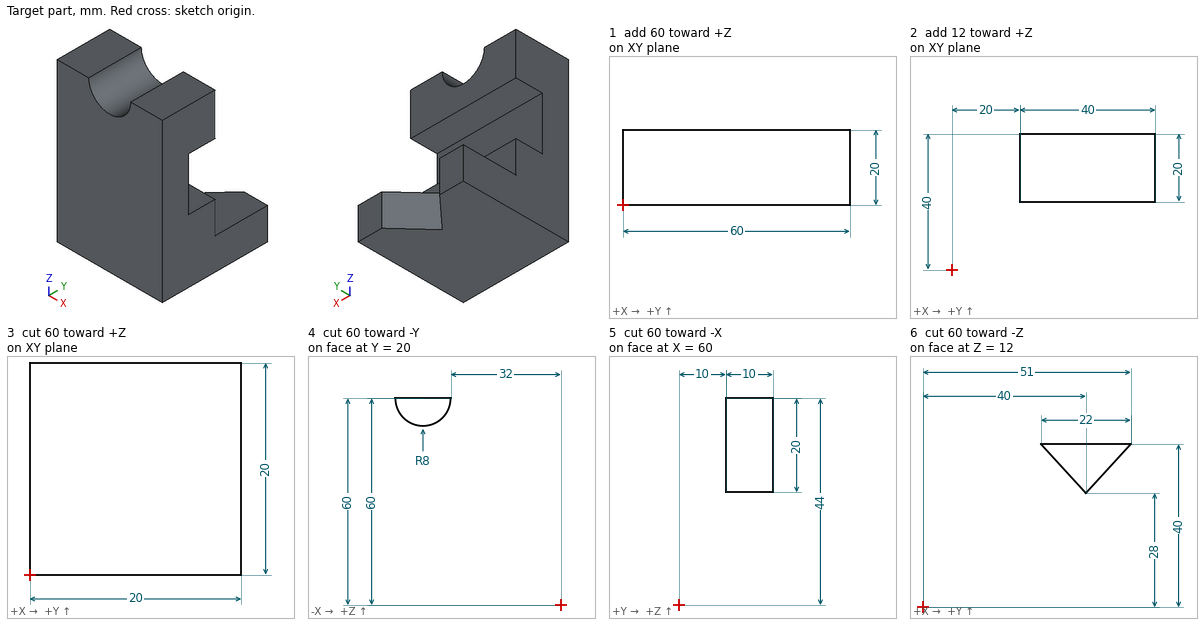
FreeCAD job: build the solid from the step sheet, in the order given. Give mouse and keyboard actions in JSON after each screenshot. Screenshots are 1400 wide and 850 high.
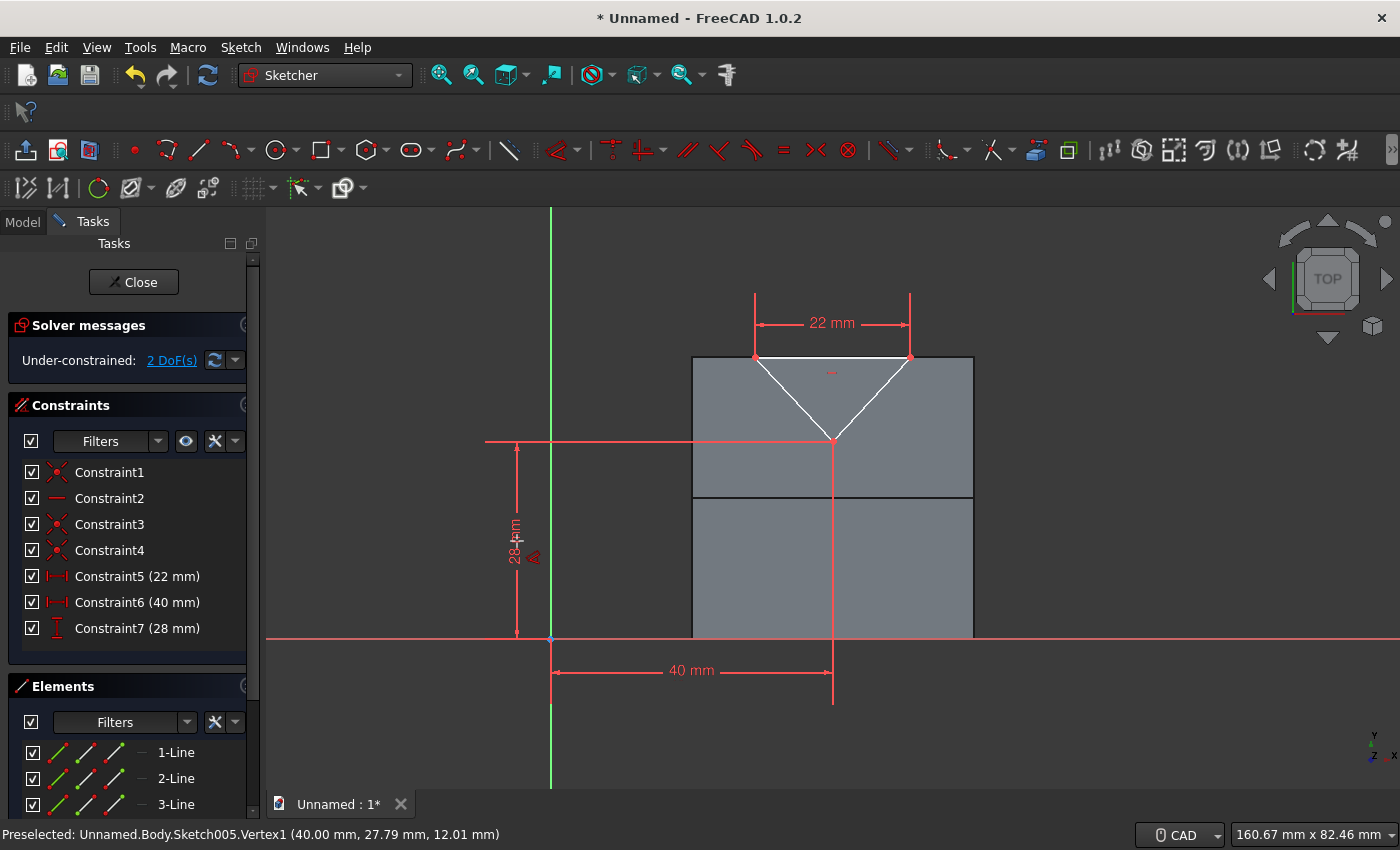
{"action": "left_click", "coordinate": [910, 358]}
{"action": "left_click", "coordinate": [813, 673]}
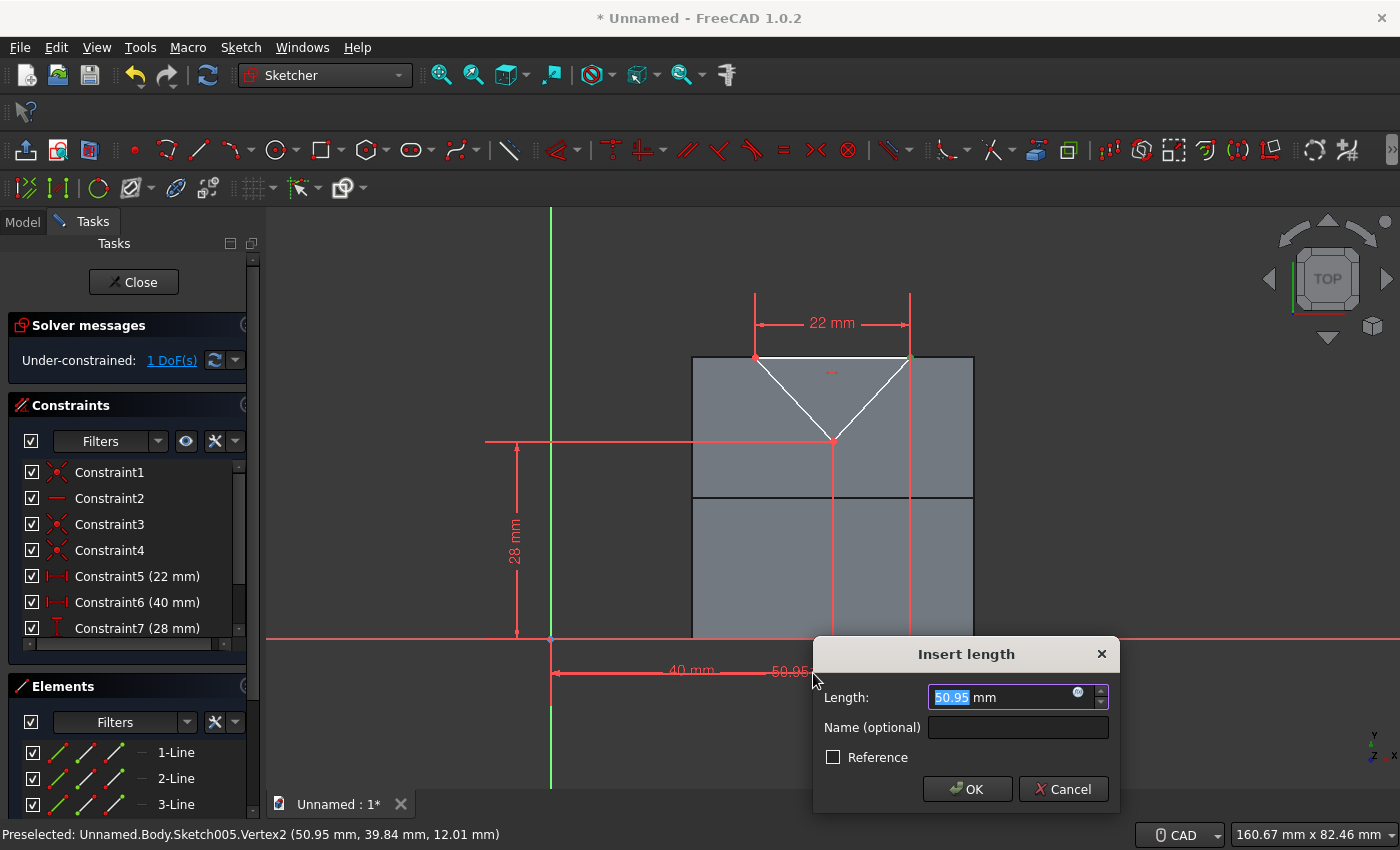
{"action": "type", "text": "51"}
{"action": "key", "text": "Return"}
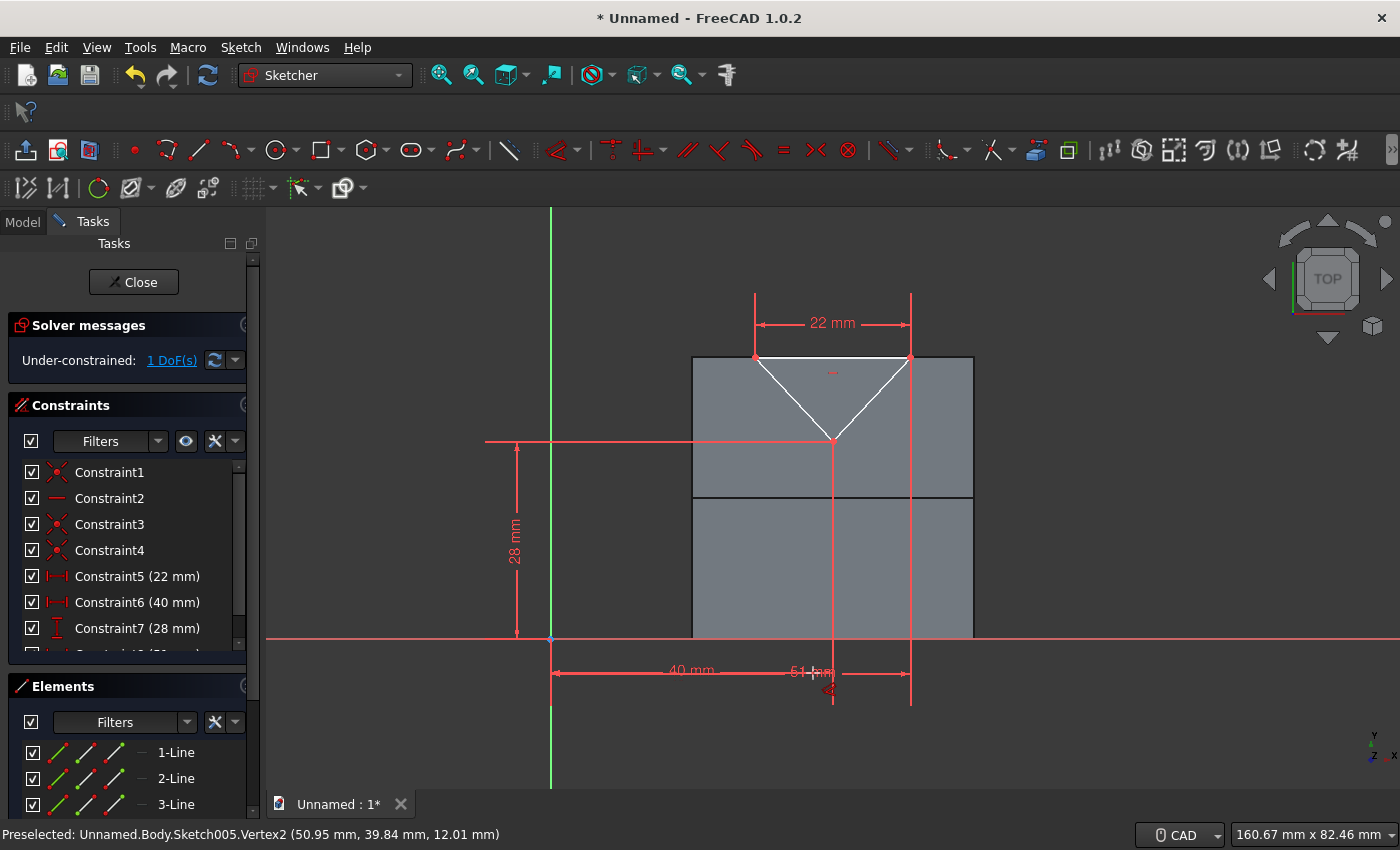
{"action": "left_click", "coordinate": [911, 358]}
{"action": "left_click", "coordinate": [945, 499]}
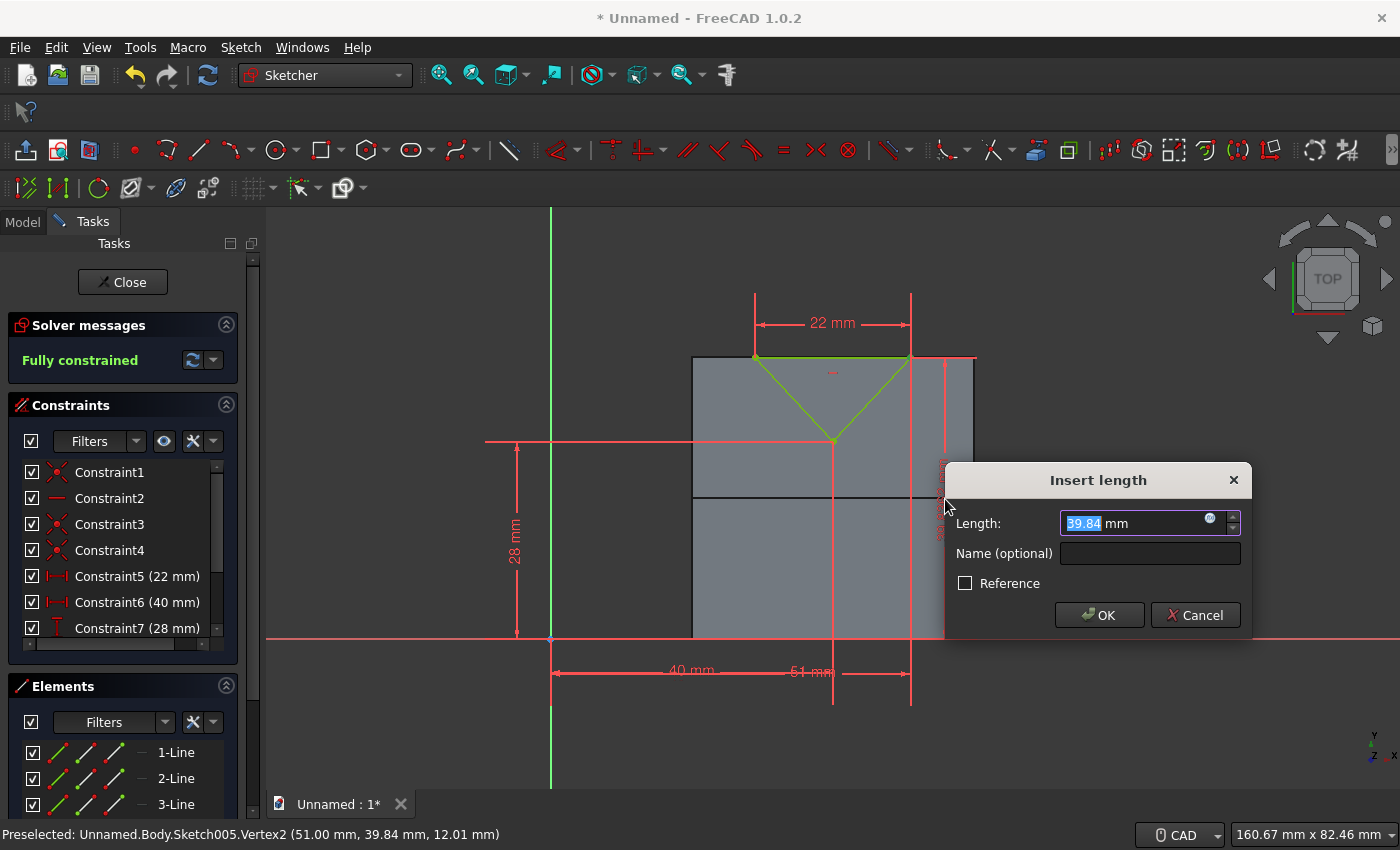
{"action": "type", "text": "40"}
{"action": "key", "text": "Return"}
{"action": "key", "text": "Escape"}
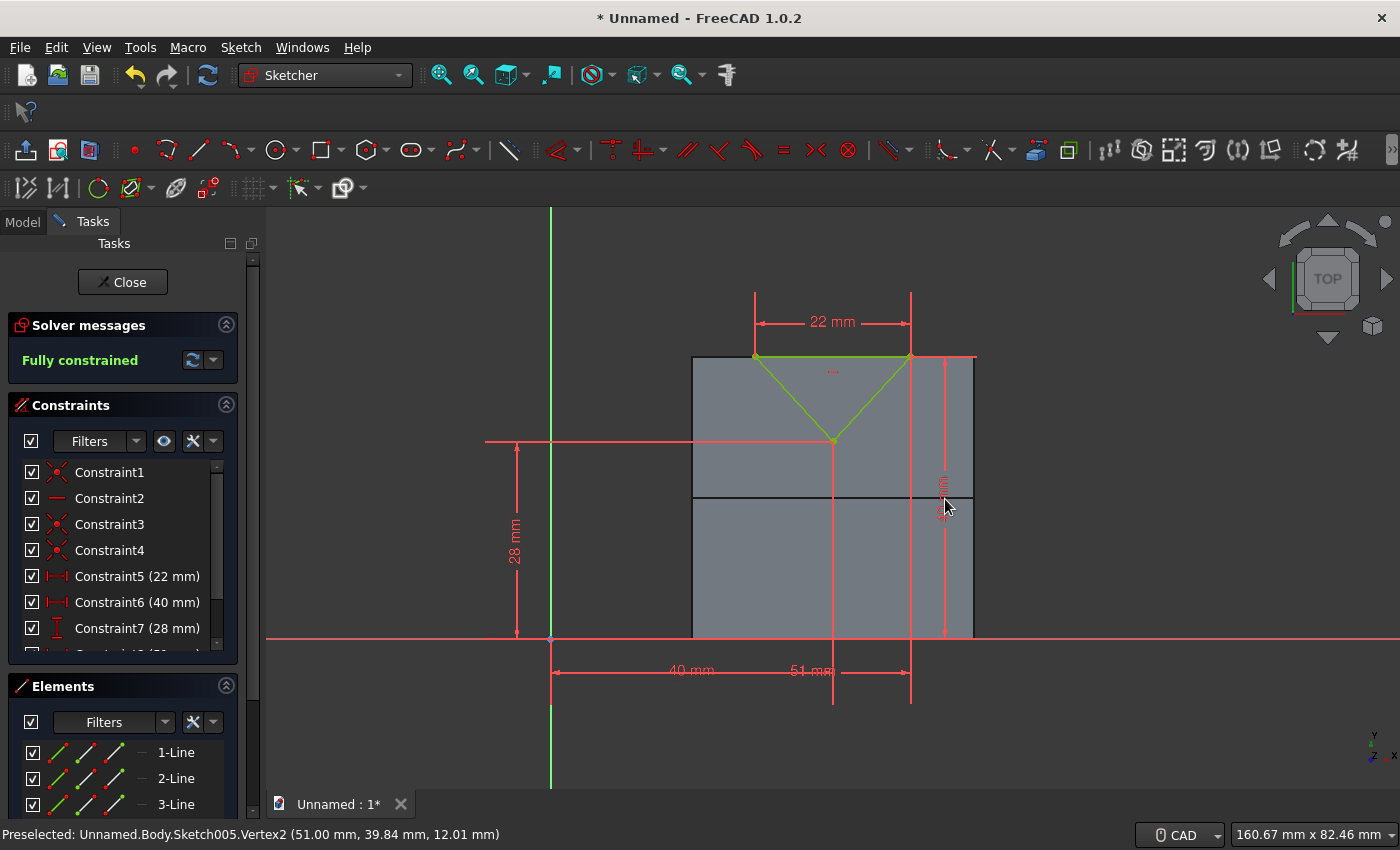
{"action": "left_click", "coordinate": [123, 282]}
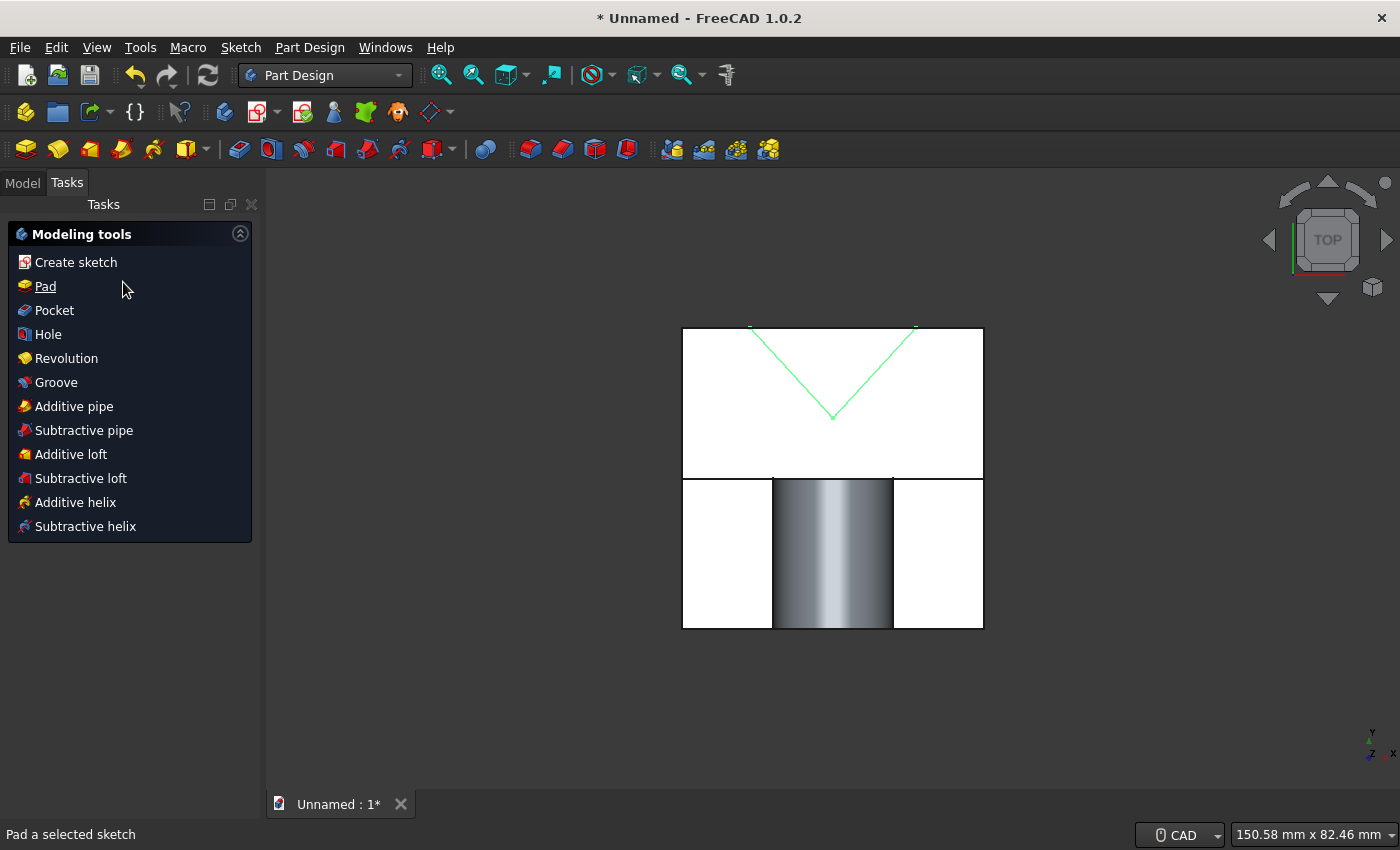
{"action": "left_click", "coordinate": [240, 150]}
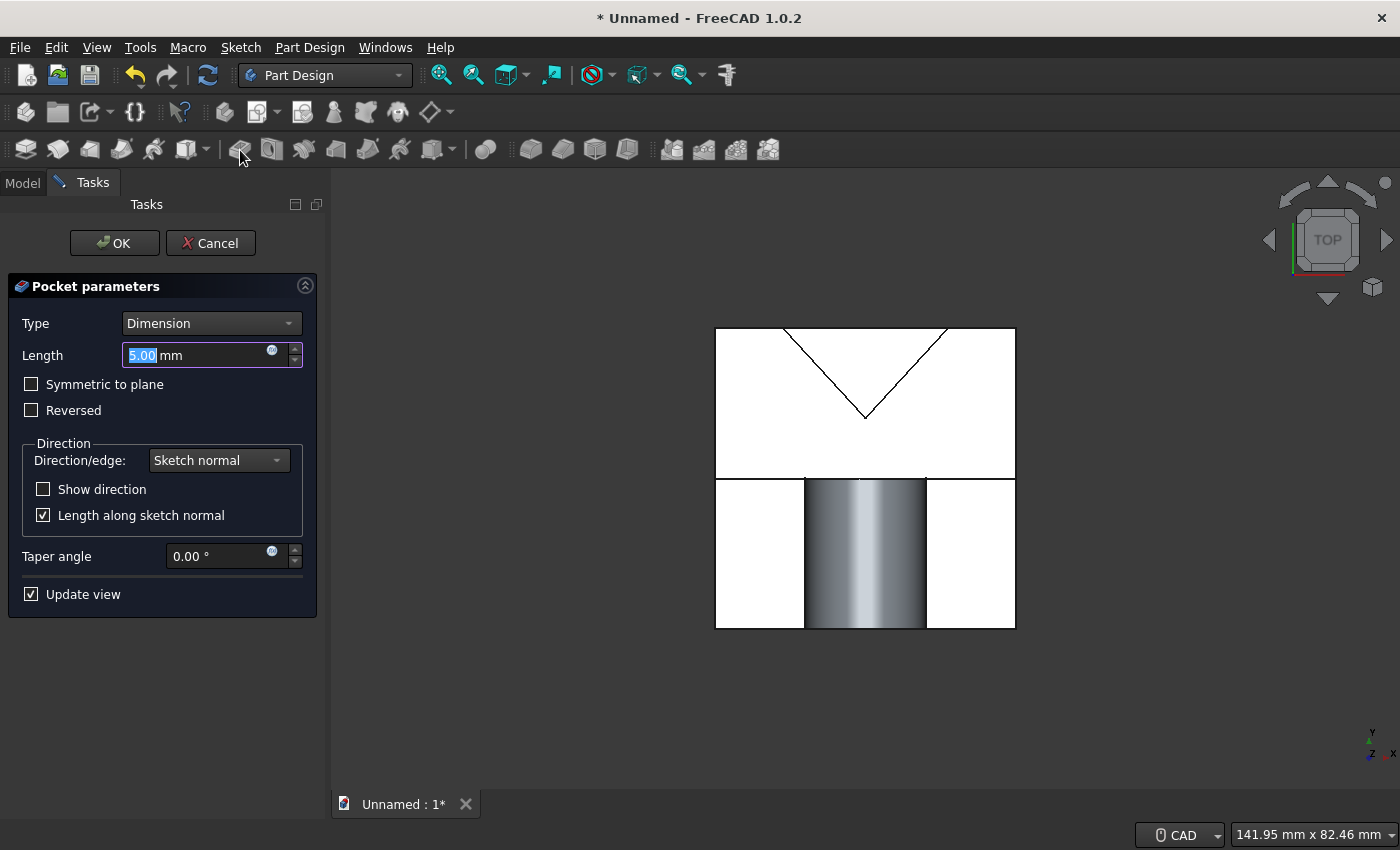
{"action": "type", "text": "60"}
{"action": "key", "text": "Tab"}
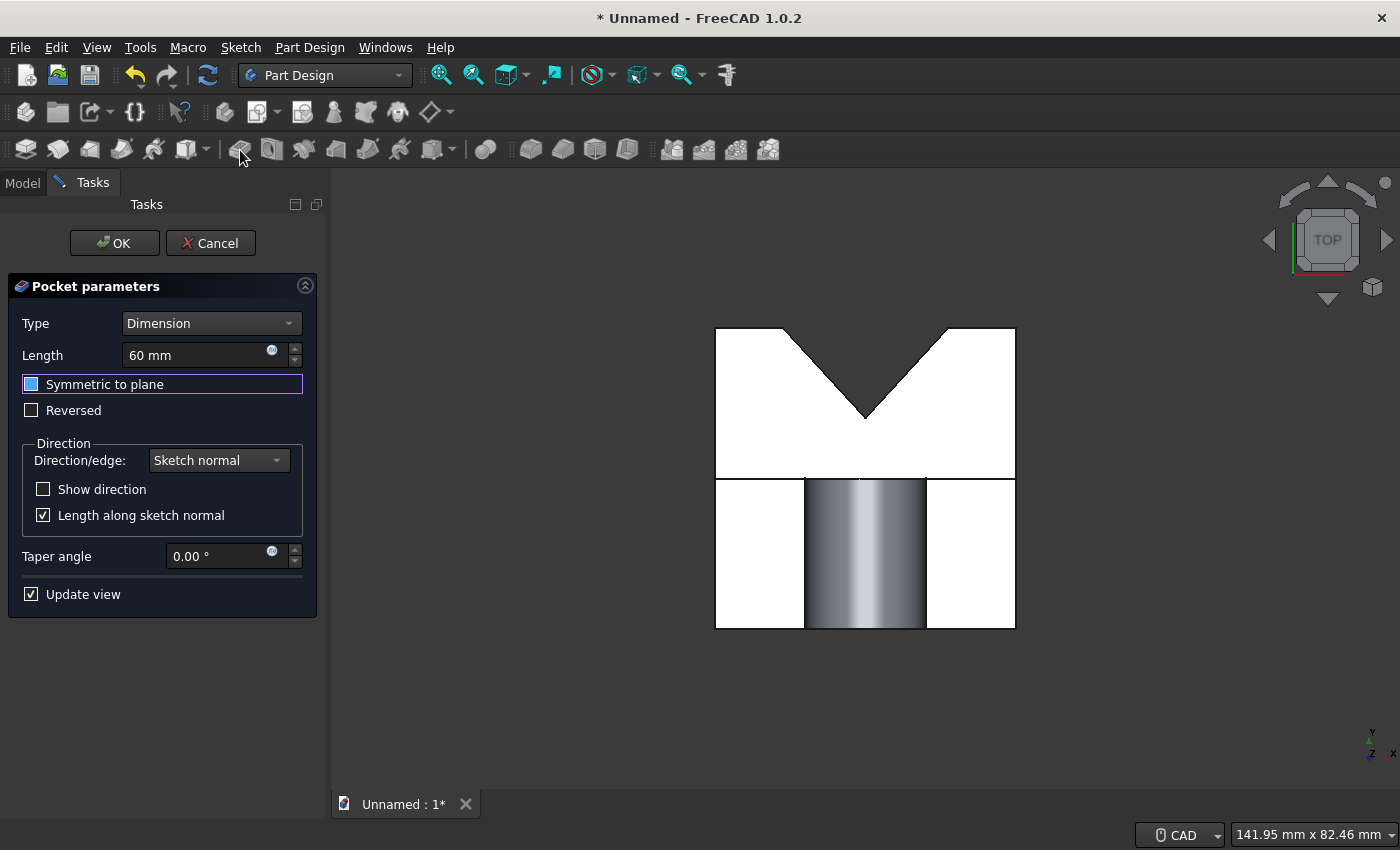
{"action": "left_click", "coordinate": [115, 243]}